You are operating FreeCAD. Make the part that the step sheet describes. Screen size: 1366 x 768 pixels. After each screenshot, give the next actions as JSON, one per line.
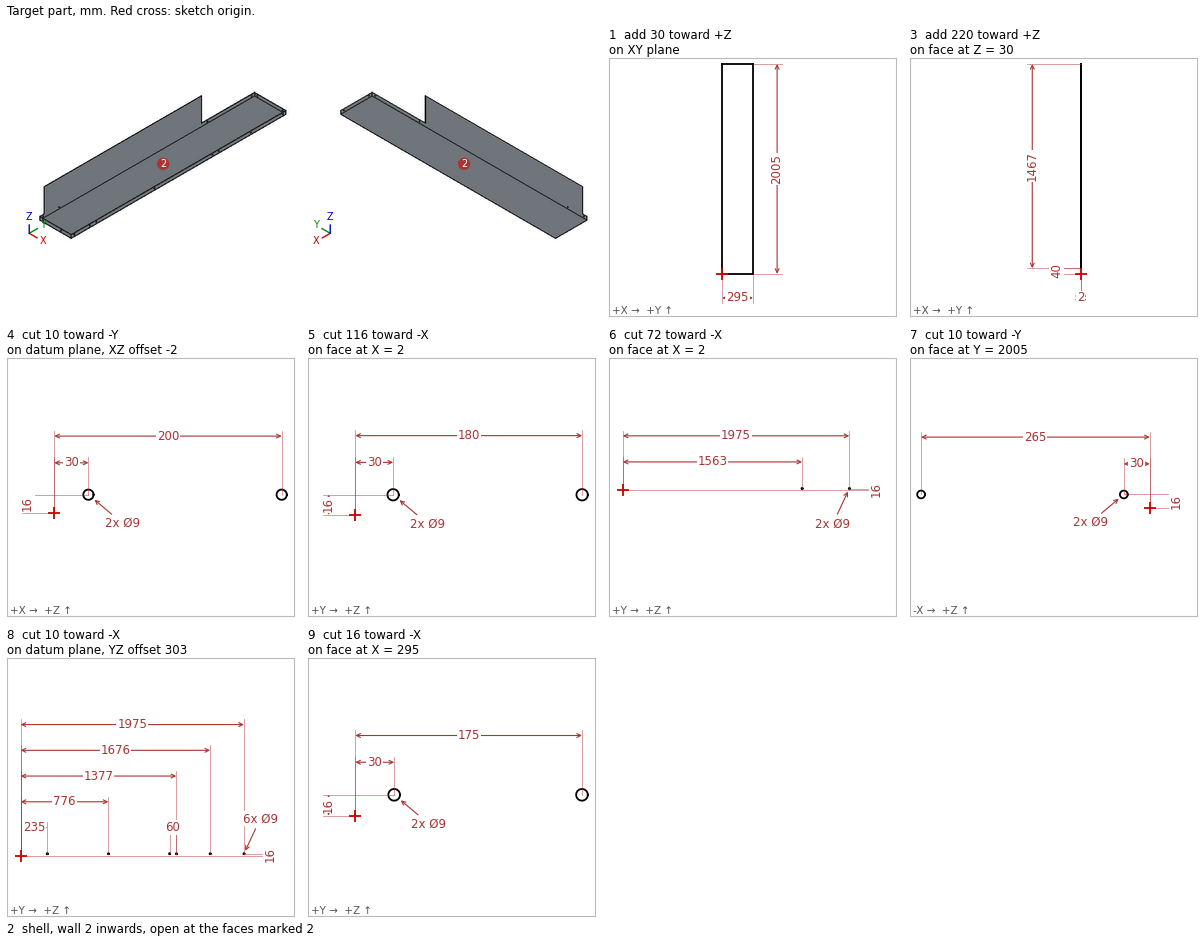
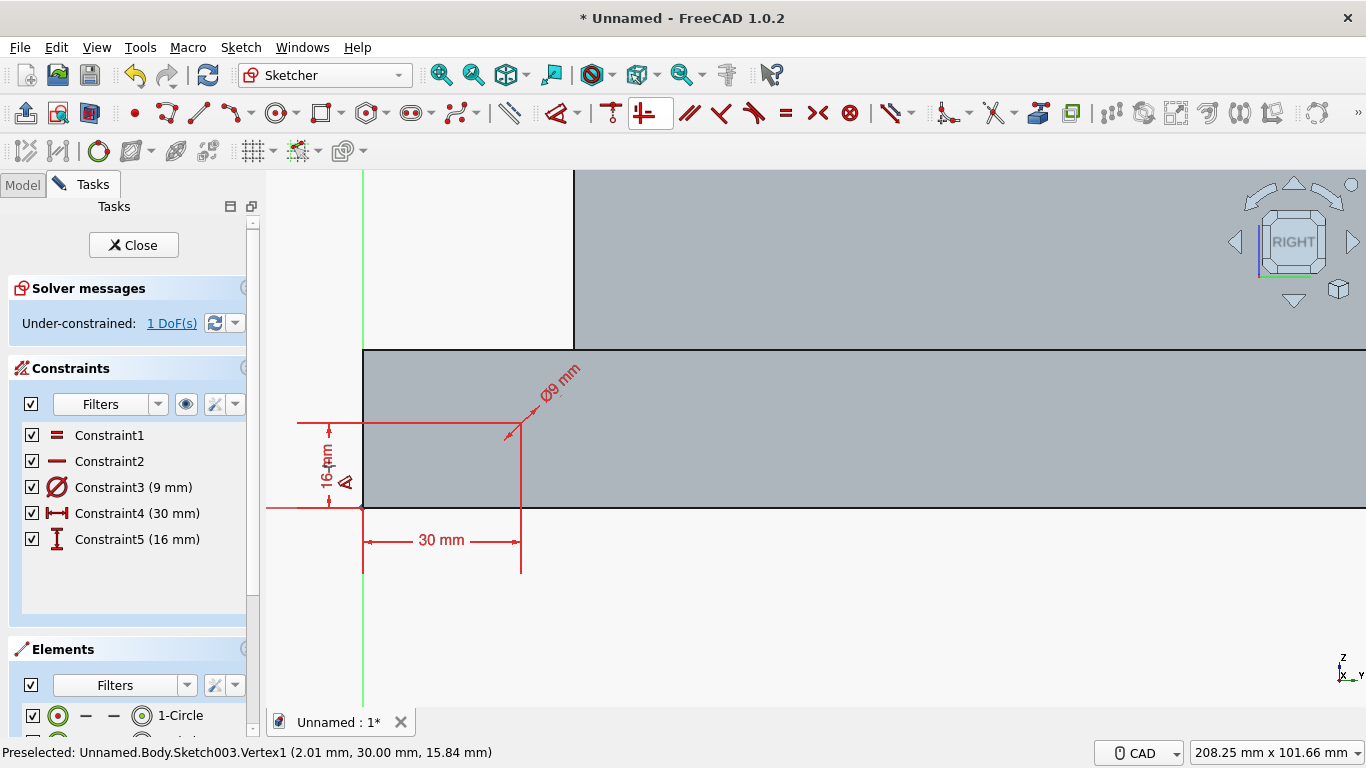
{"action": "scroll", "coordinate": [539, 407], "scroll_direction": "down", "scroll_amount": 2}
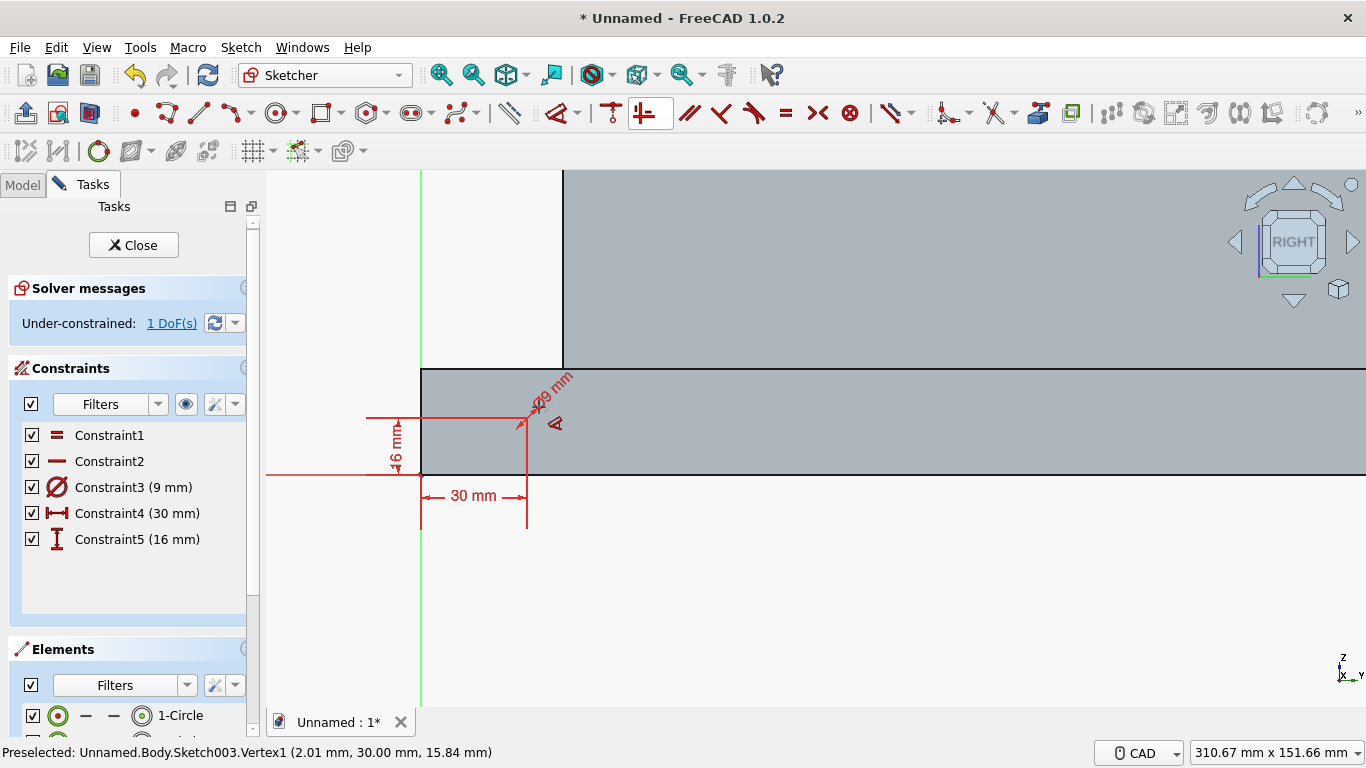
{"action": "left_click", "coordinate": [1058, 418]}
{"action": "left_click", "coordinate": [740, 509]}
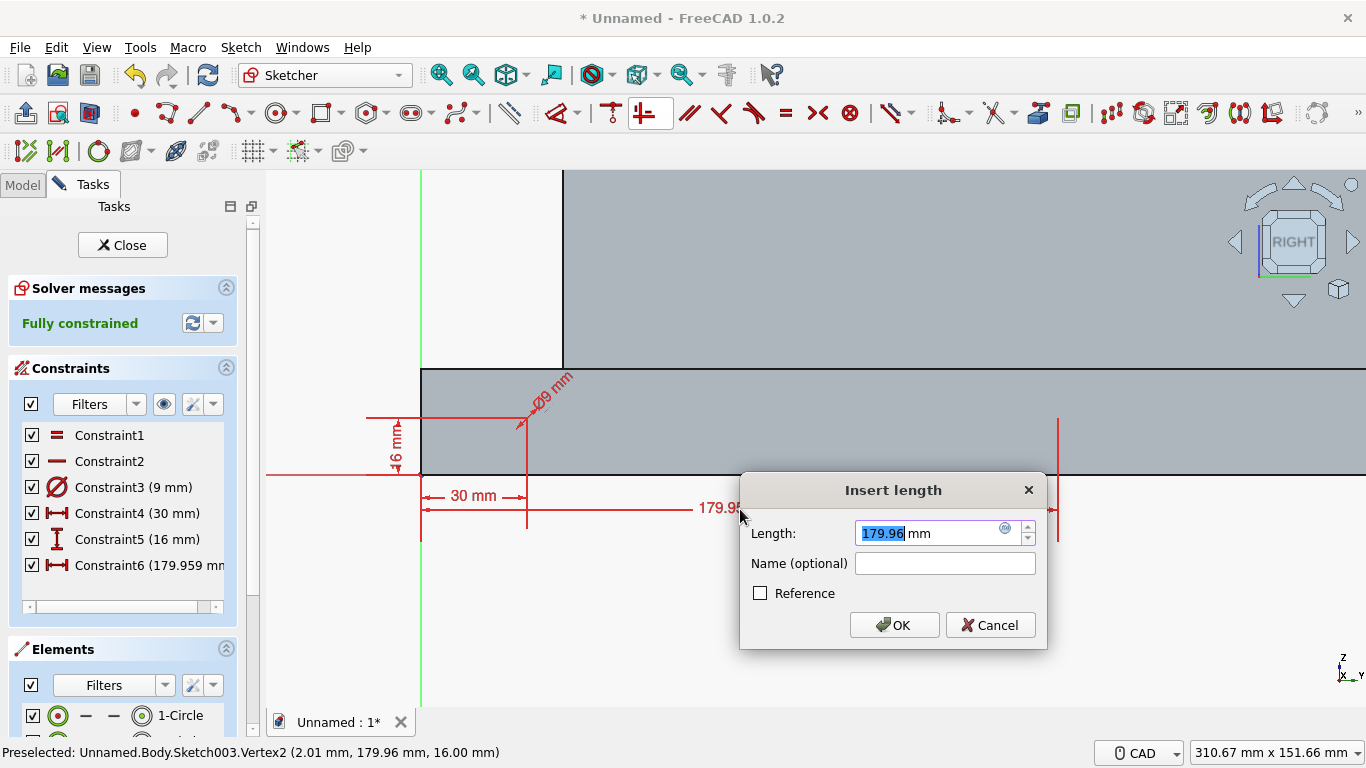
{"action": "type", "text": "180"}
{"action": "key", "text": "Return"}
{"action": "key", "text": "Escape"}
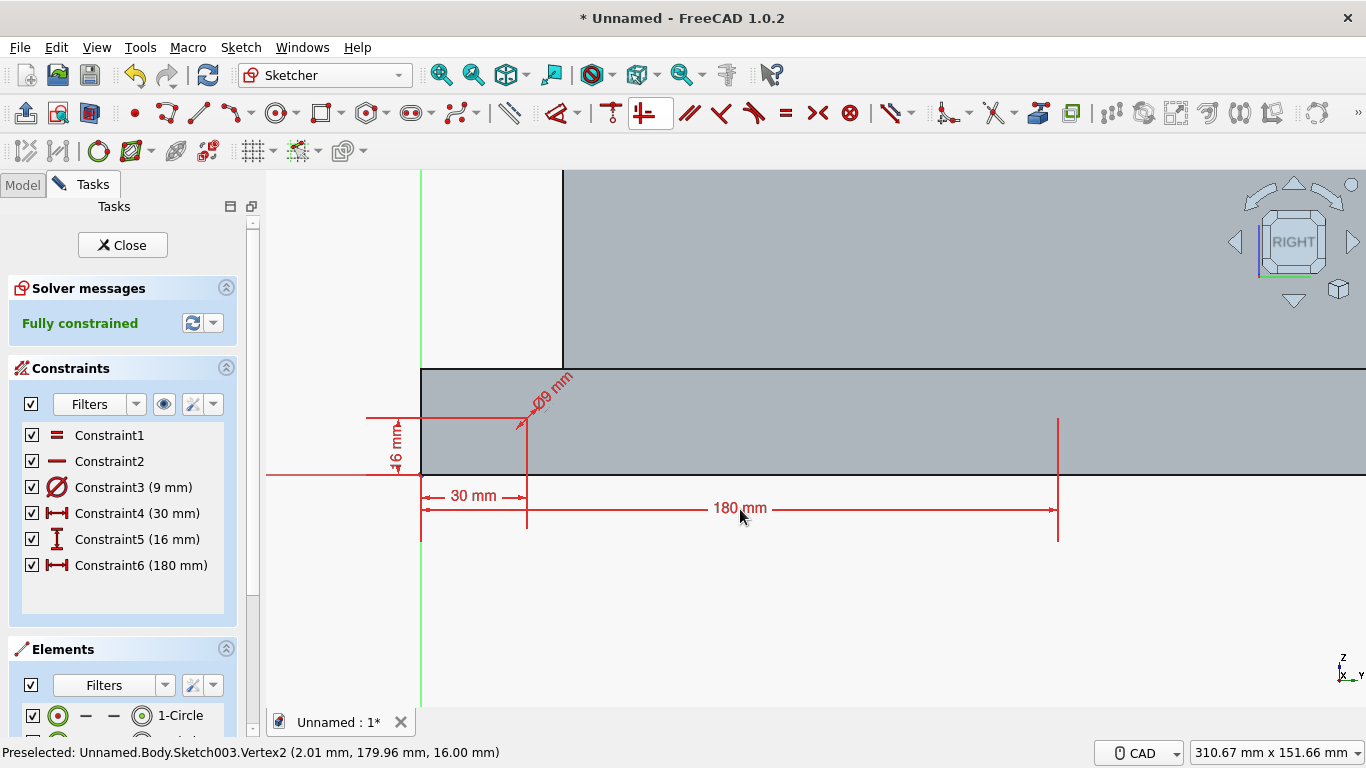
{"action": "left_click", "coordinate": [123, 245]}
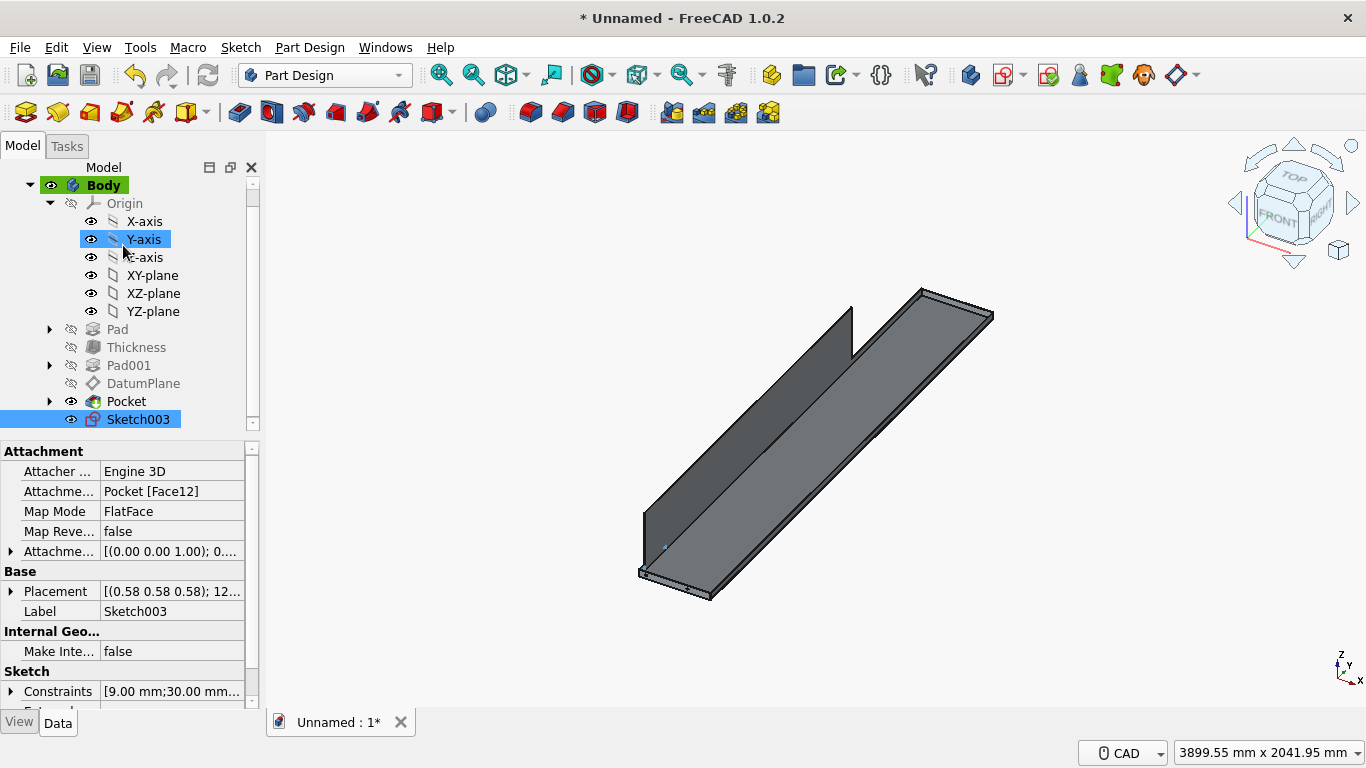
{"action": "left_click", "coordinate": [240, 112]}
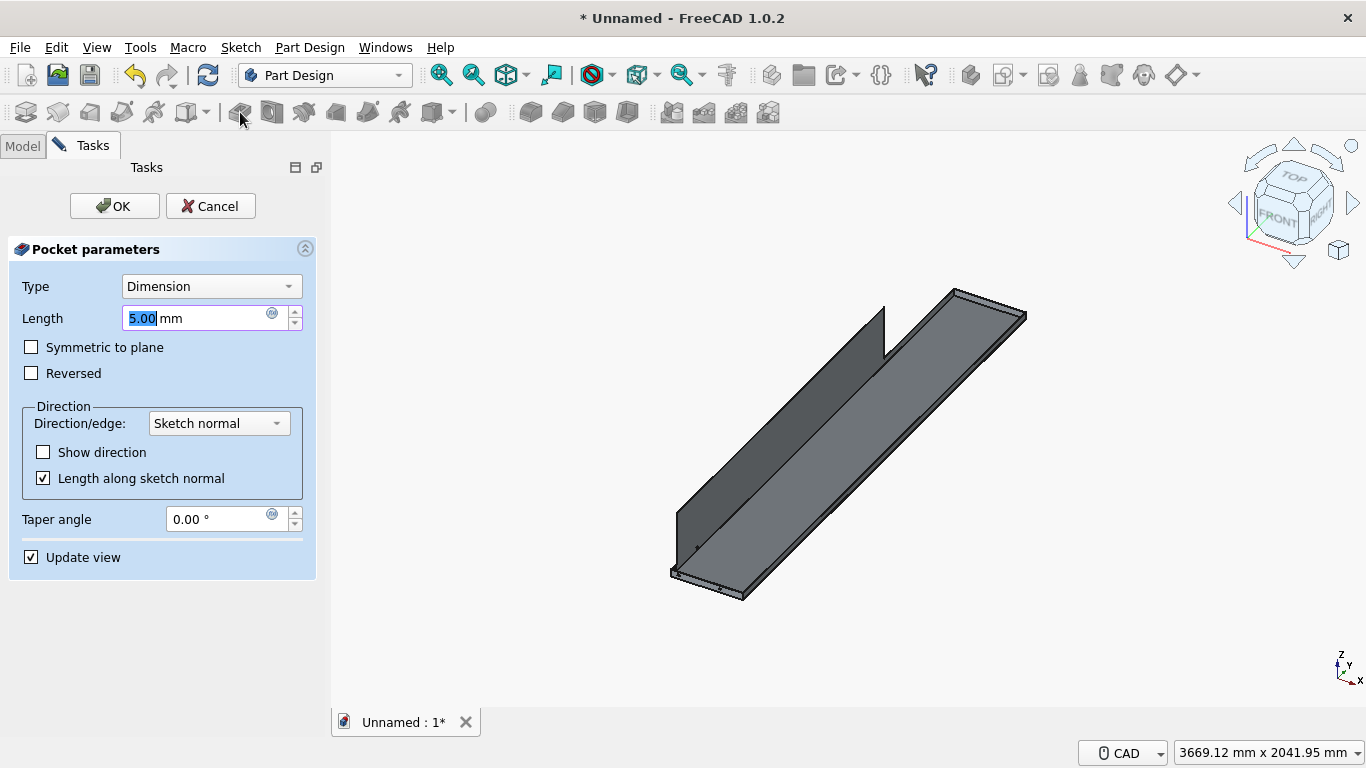
{"action": "type", "text": "116"}
{"action": "key", "text": "Tab"}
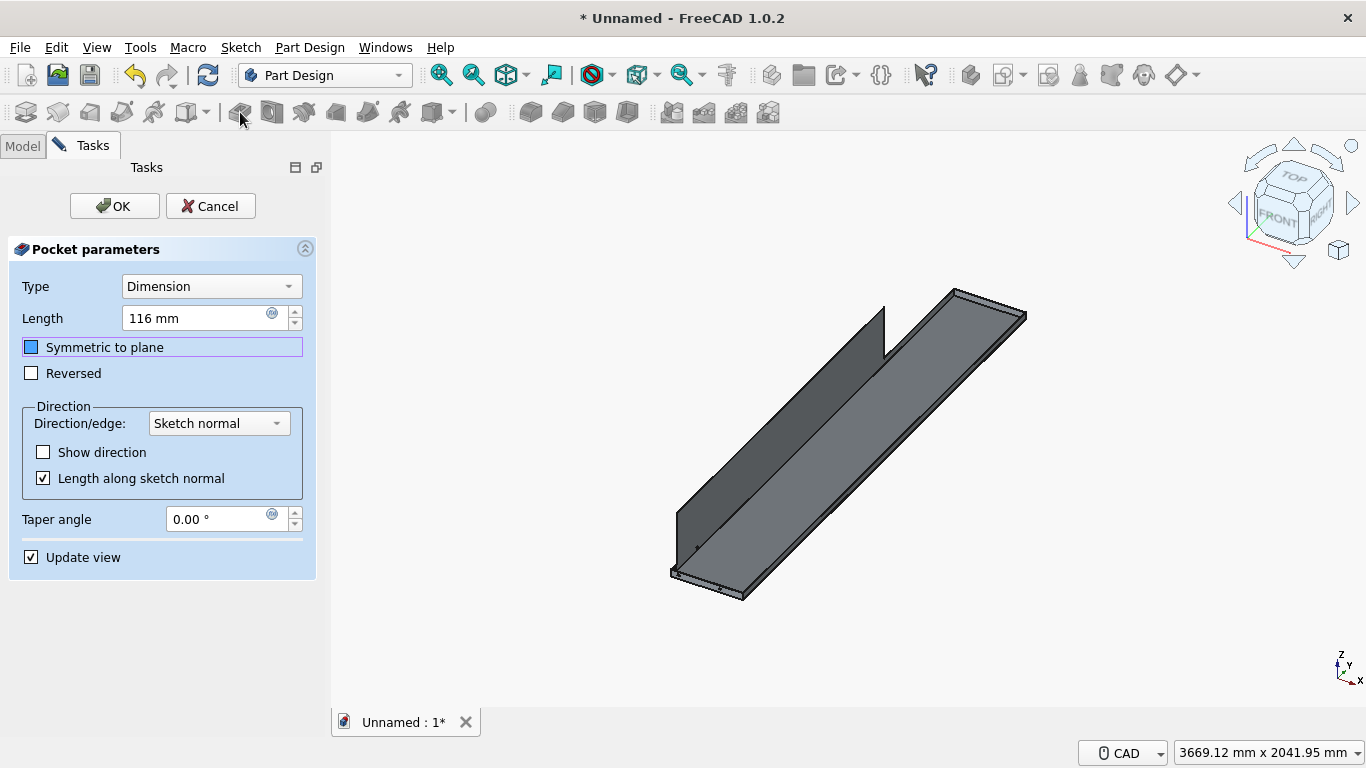
{"action": "left_click", "coordinate": [115, 206]}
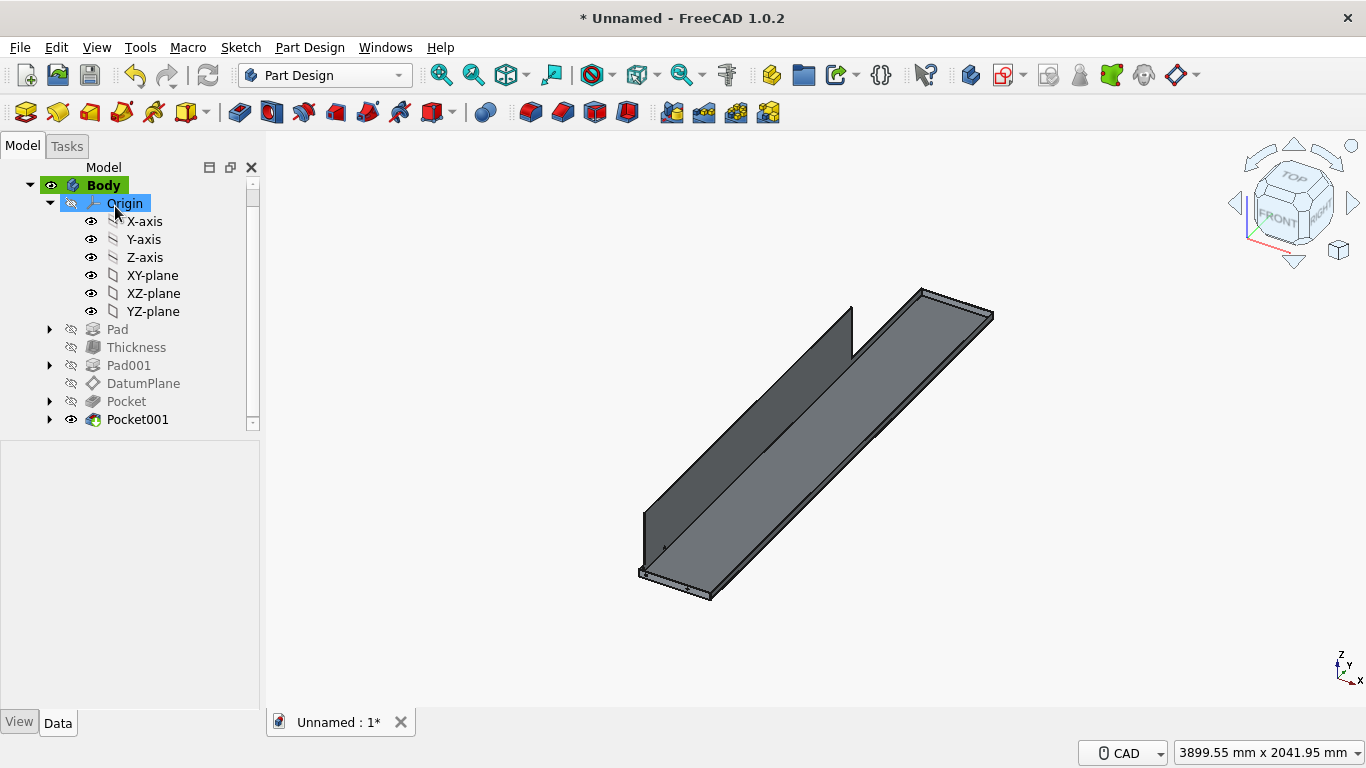
{"action": "left_click", "coordinate": [821, 366]}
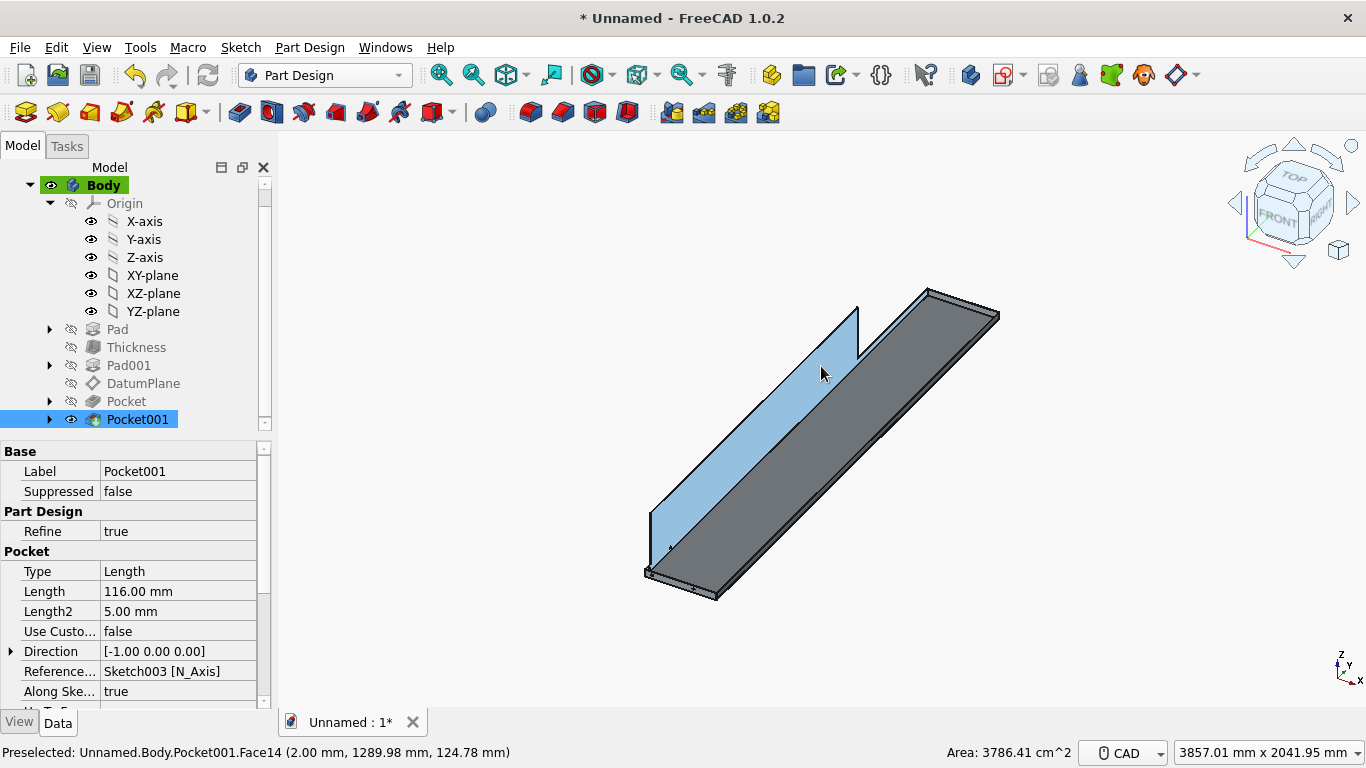
{"action": "left_click", "coordinate": [1004, 76]}